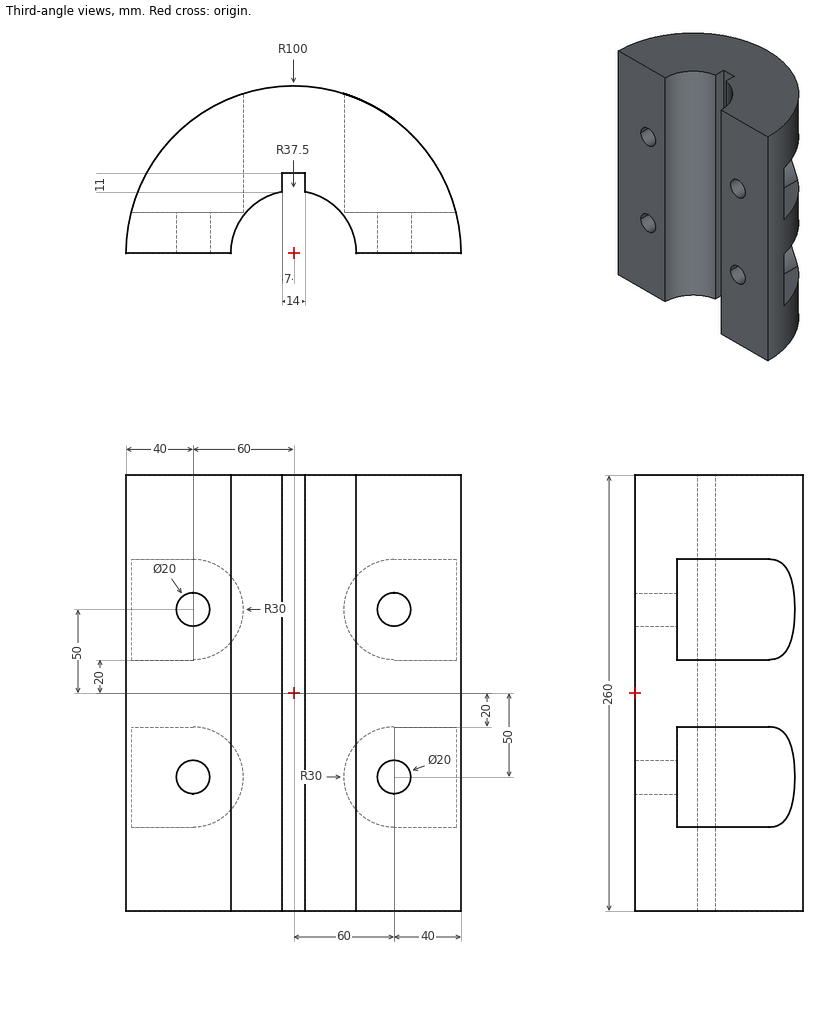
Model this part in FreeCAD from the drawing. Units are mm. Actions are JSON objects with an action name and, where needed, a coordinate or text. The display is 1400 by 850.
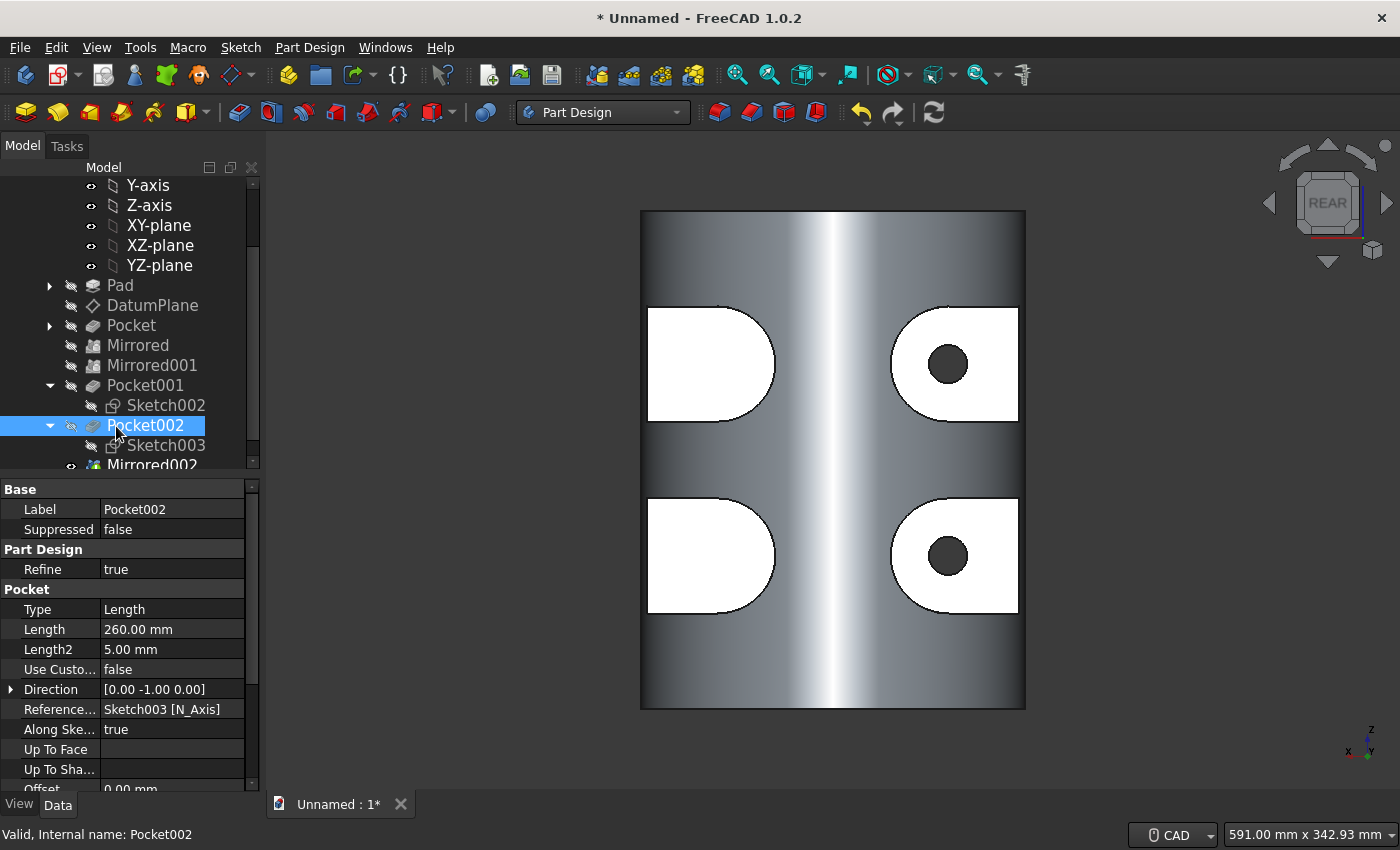
{"action": "left_click", "coordinate": [598, 76]}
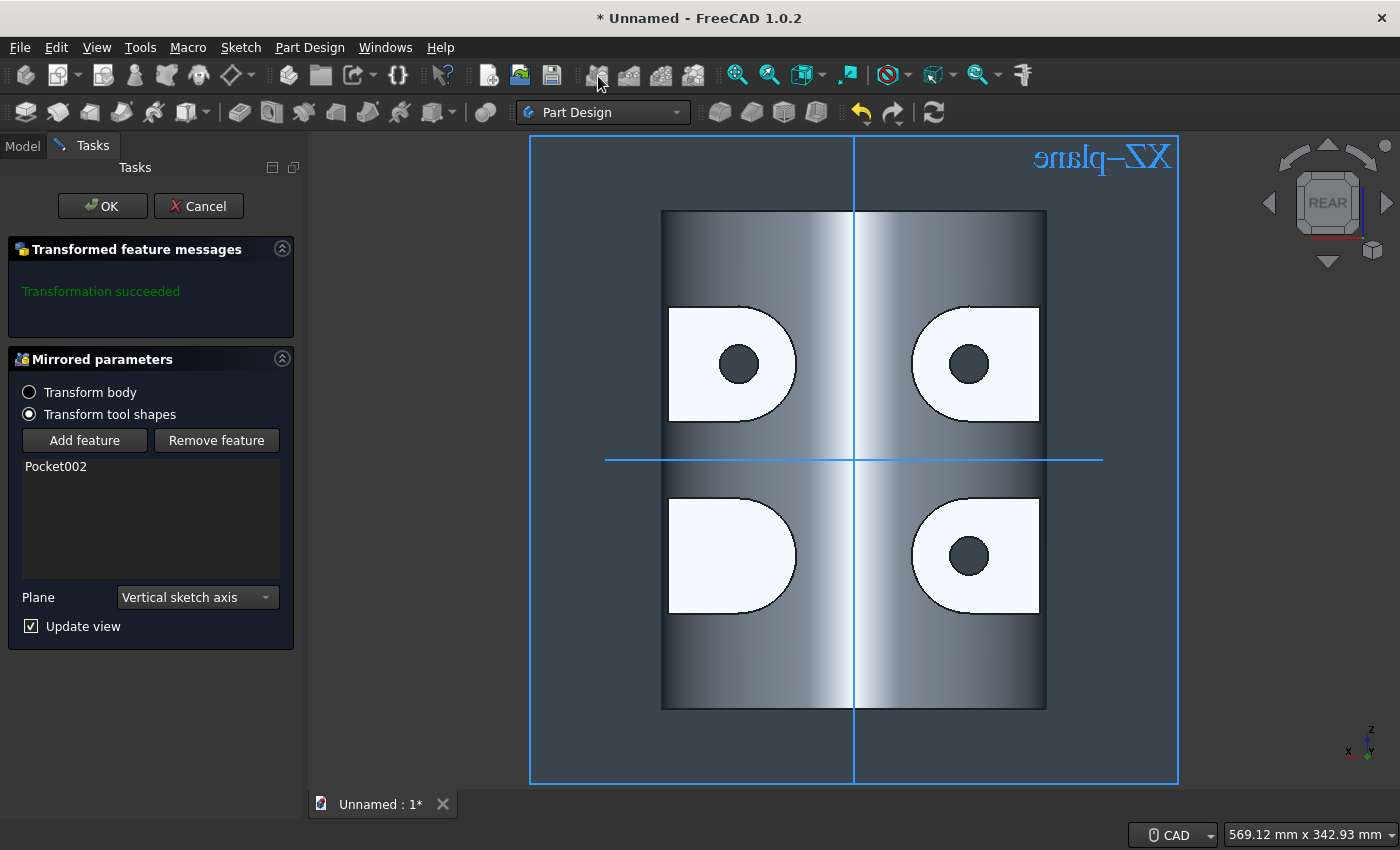
{"action": "left_click", "coordinate": [198, 598]}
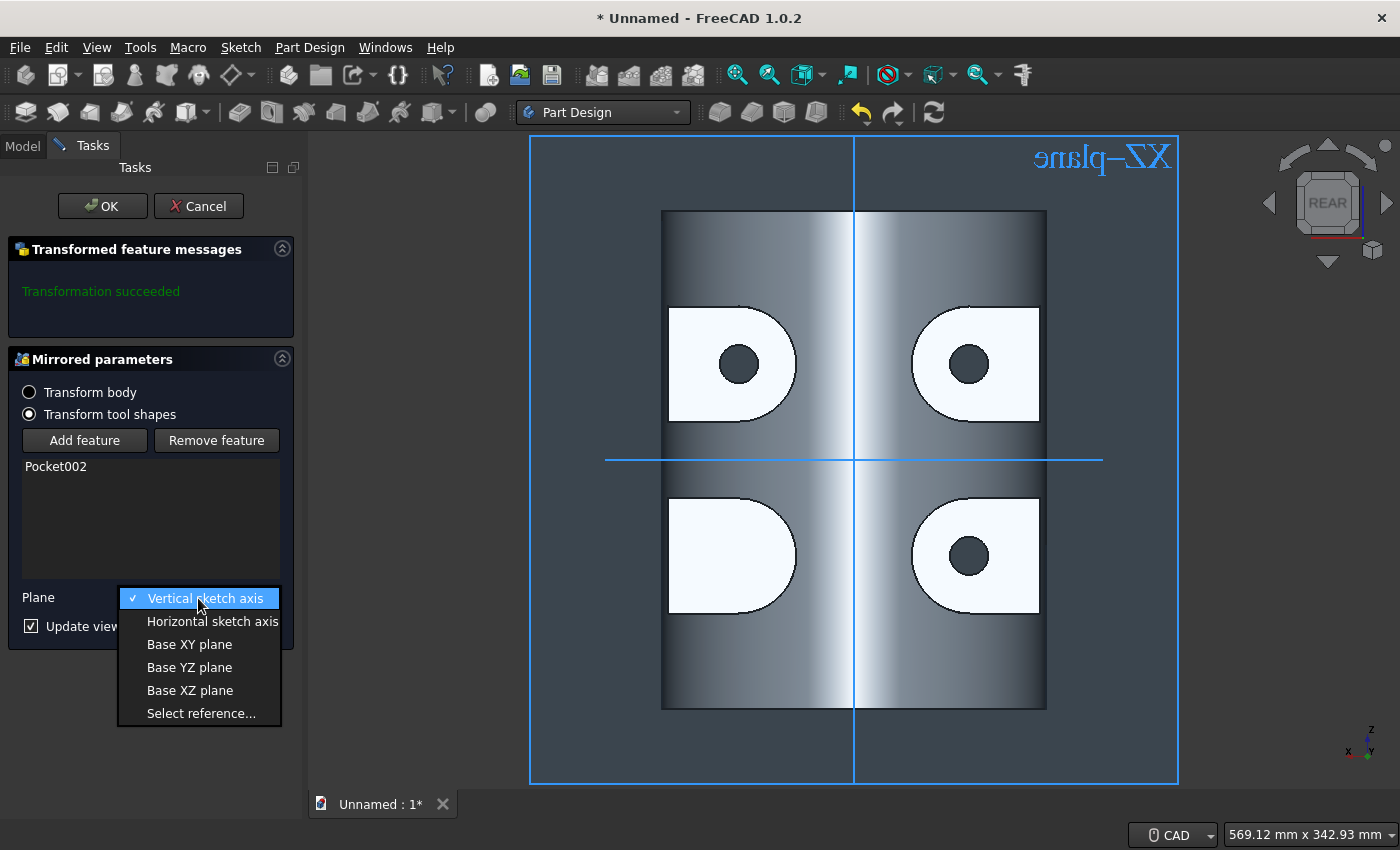
{"action": "left_click", "coordinate": [198, 668]}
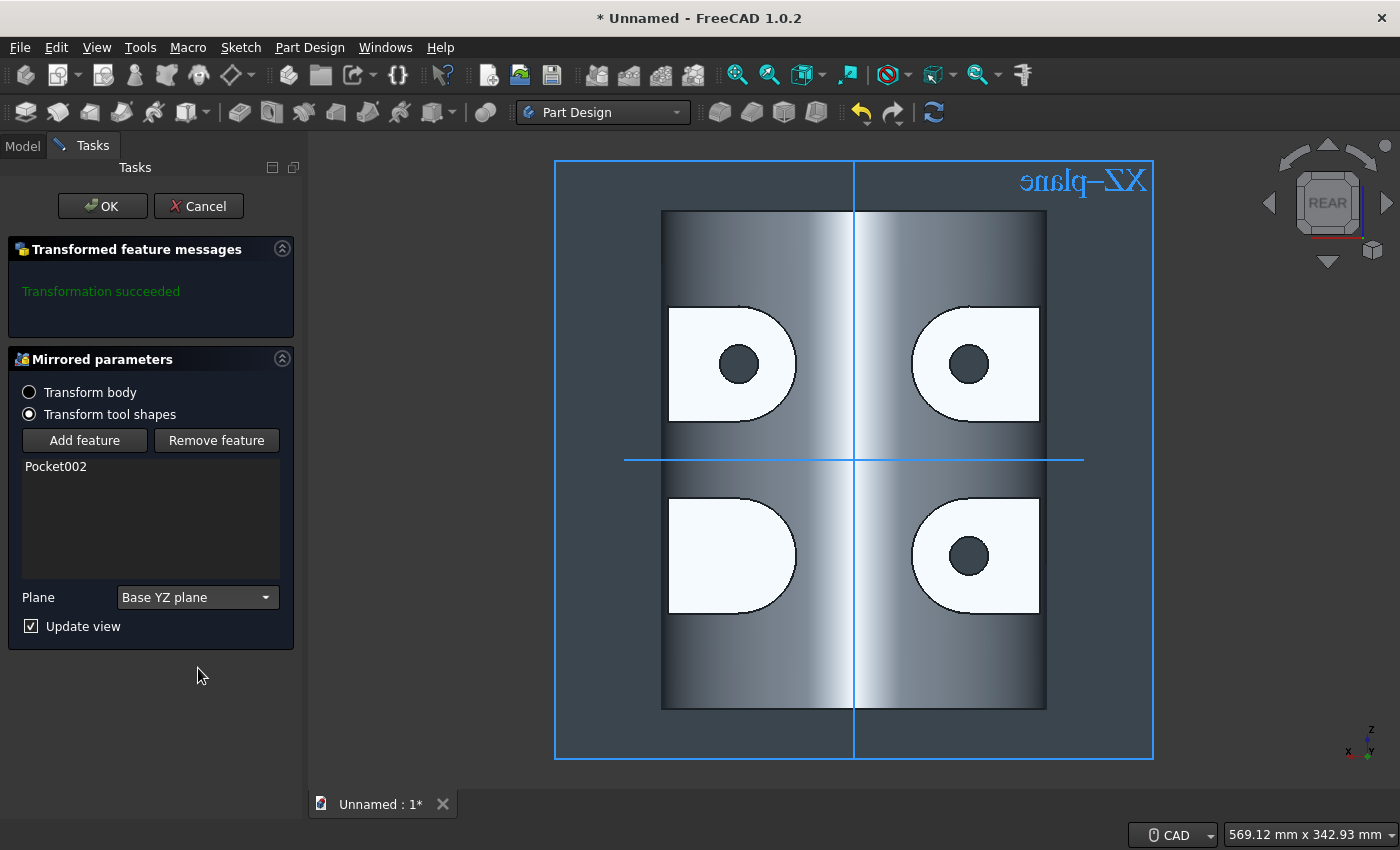
{"action": "left_click", "coordinate": [103, 206]}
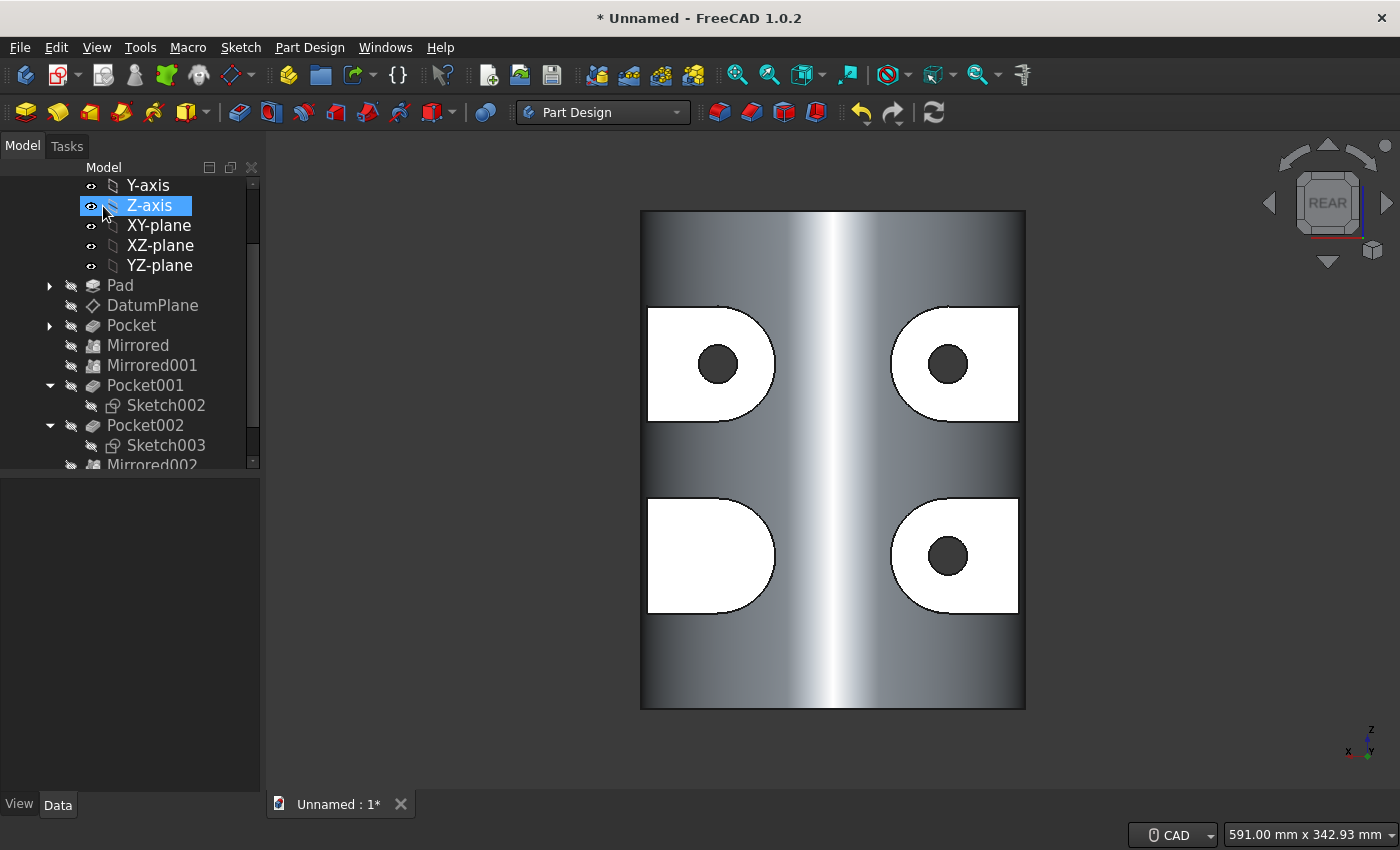
{"action": "left_click", "coordinate": [711, 555]}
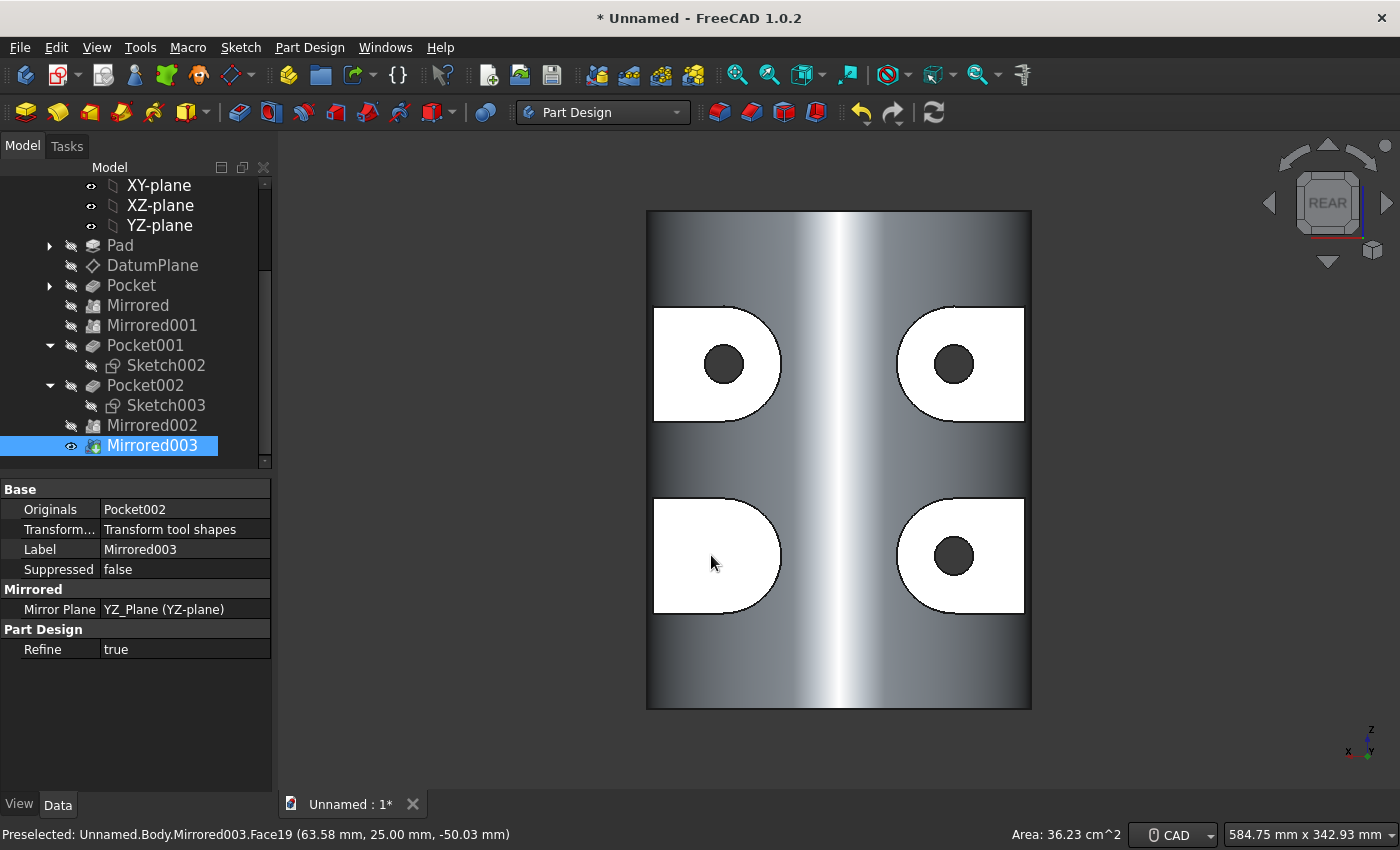
{"action": "left_click", "coordinate": [58, 76]}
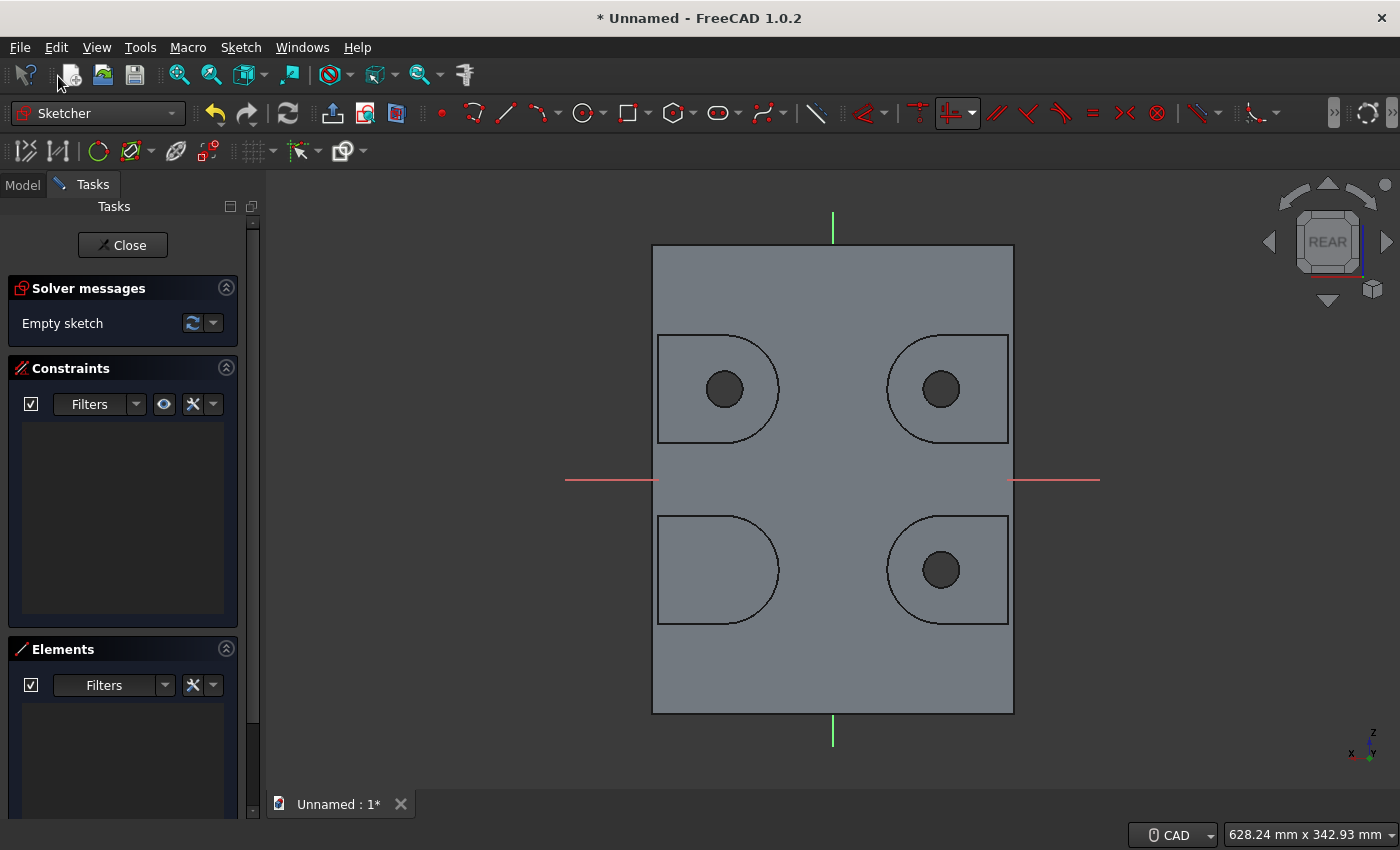
{"action": "scroll", "coordinate": [721, 579], "scroll_direction": "up", "scroll_amount": 12}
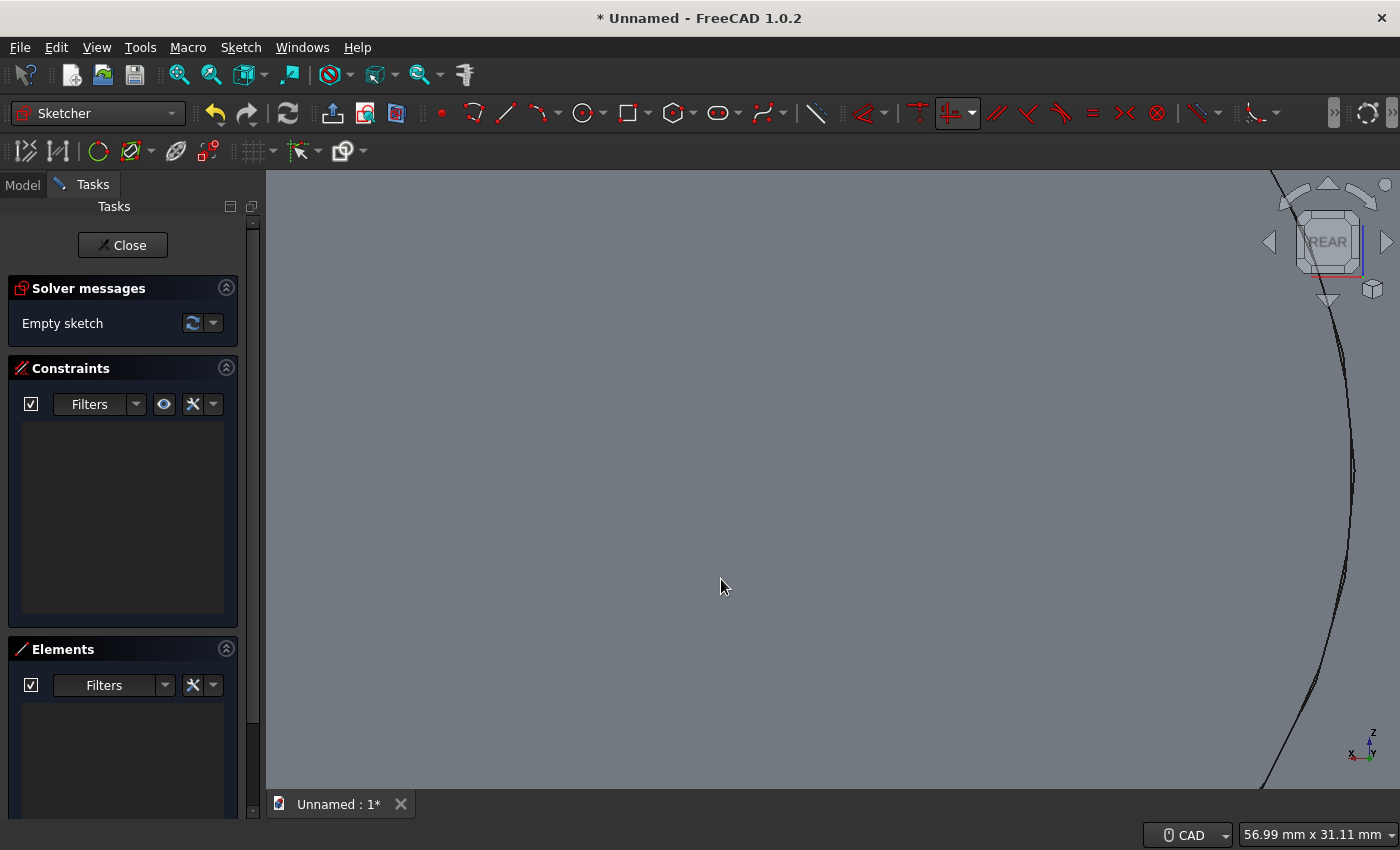
{"action": "left_click", "coordinate": [584, 114]}